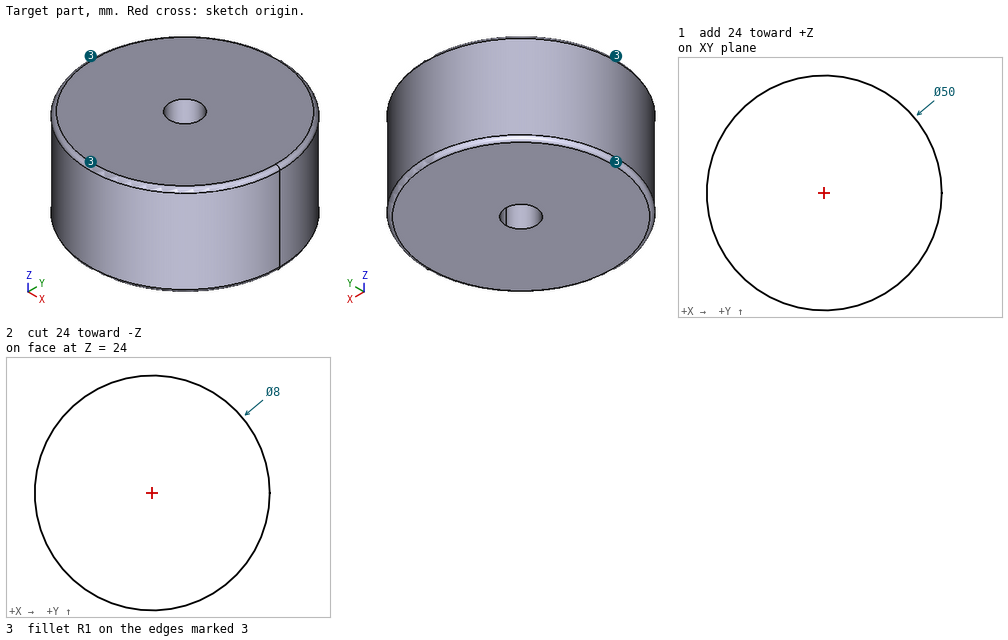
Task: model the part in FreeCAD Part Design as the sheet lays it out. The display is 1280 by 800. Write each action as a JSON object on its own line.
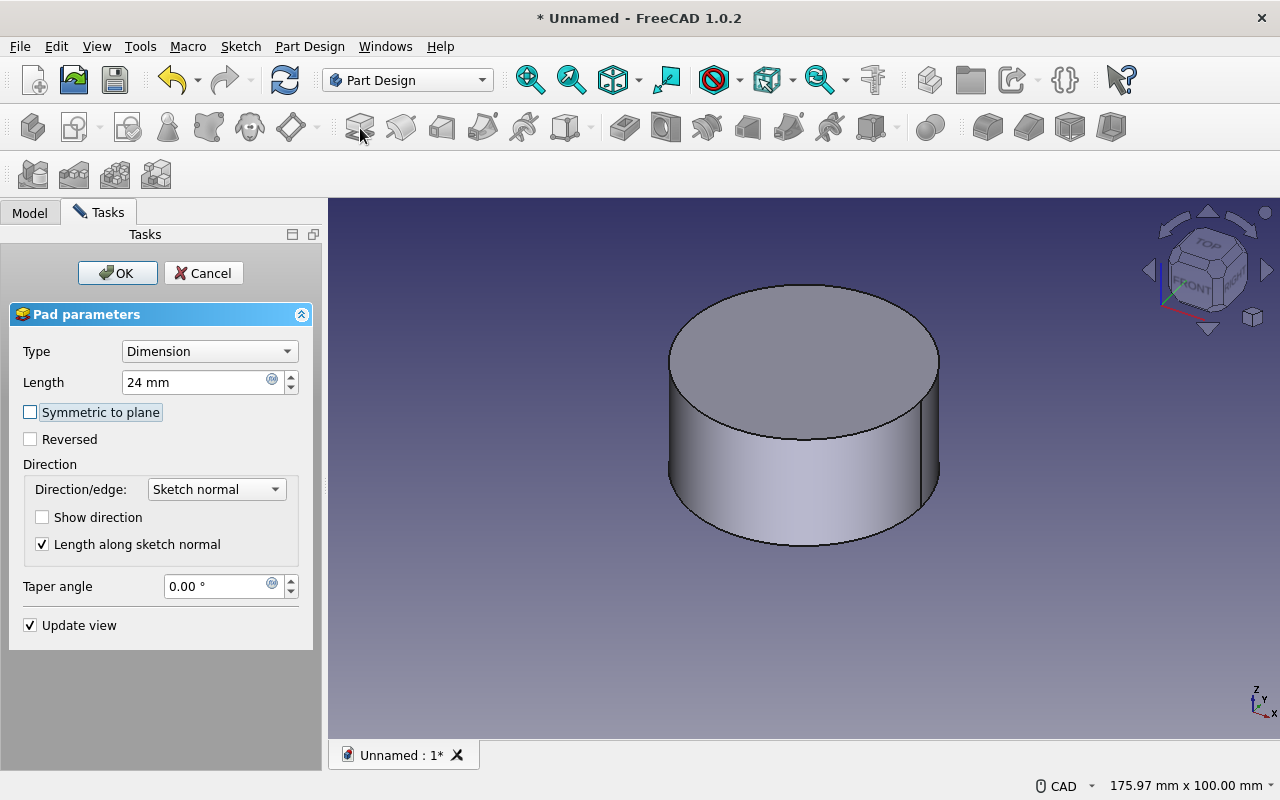
{"action": "left_click", "coordinate": [118, 273]}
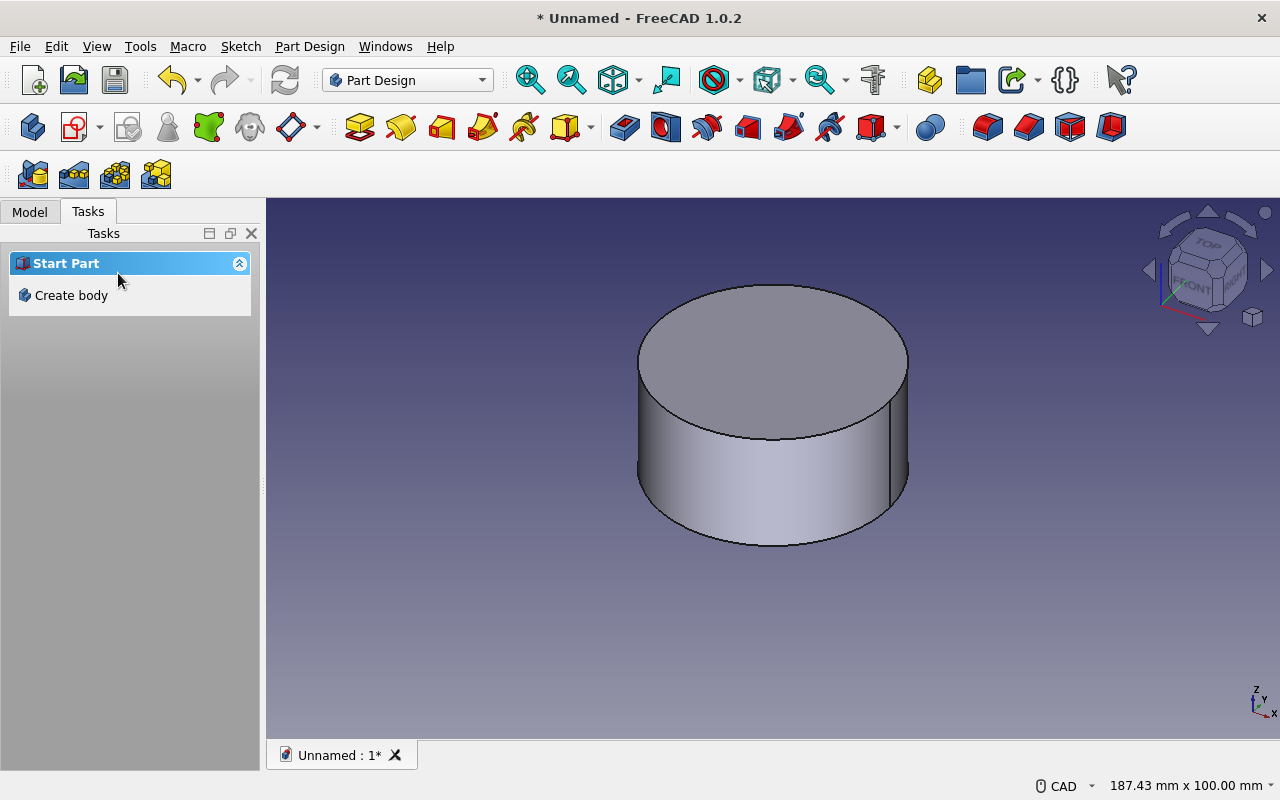
{"action": "left_click", "coordinate": [773, 361]}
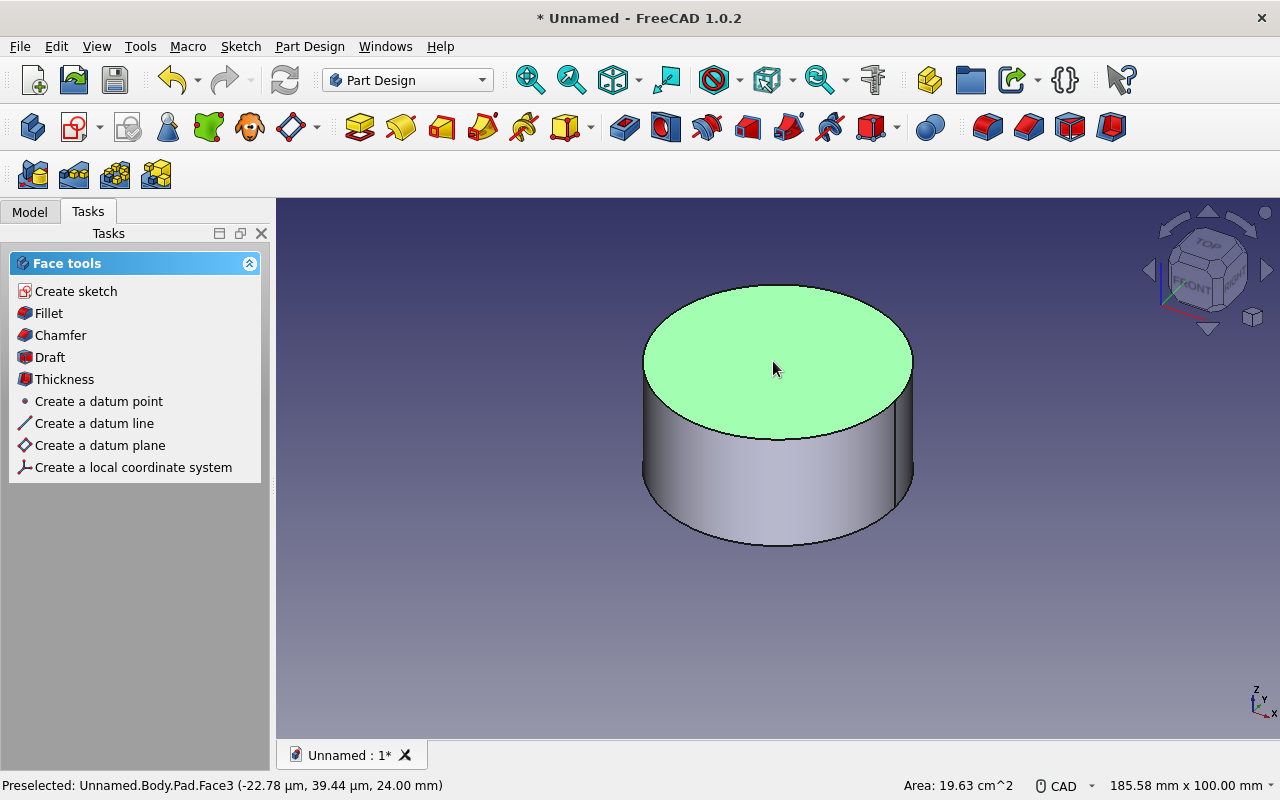
{"action": "left_click", "coordinate": [74, 128]}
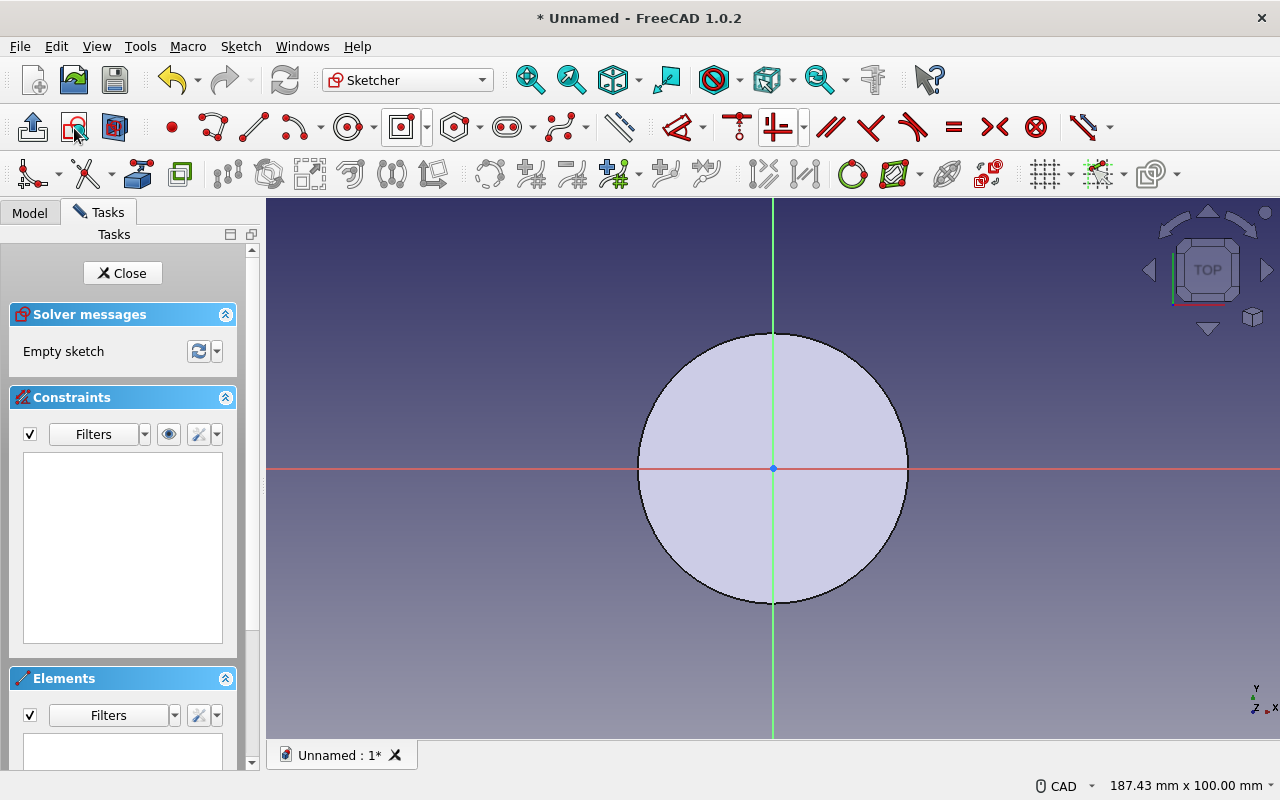
{"action": "scroll", "coordinate": [784, 468], "scroll_direction": "up", "scroll_amount": 10}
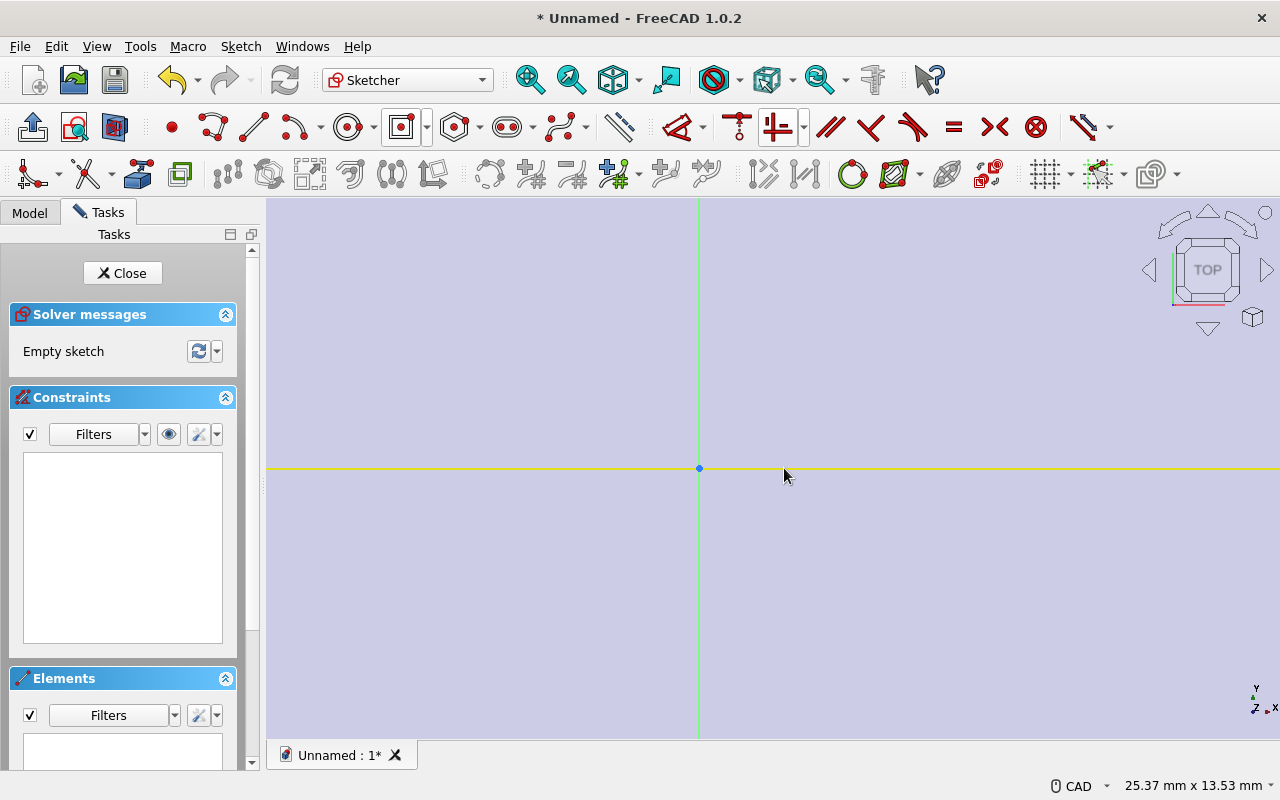
{"action": "key", "text": "g c"}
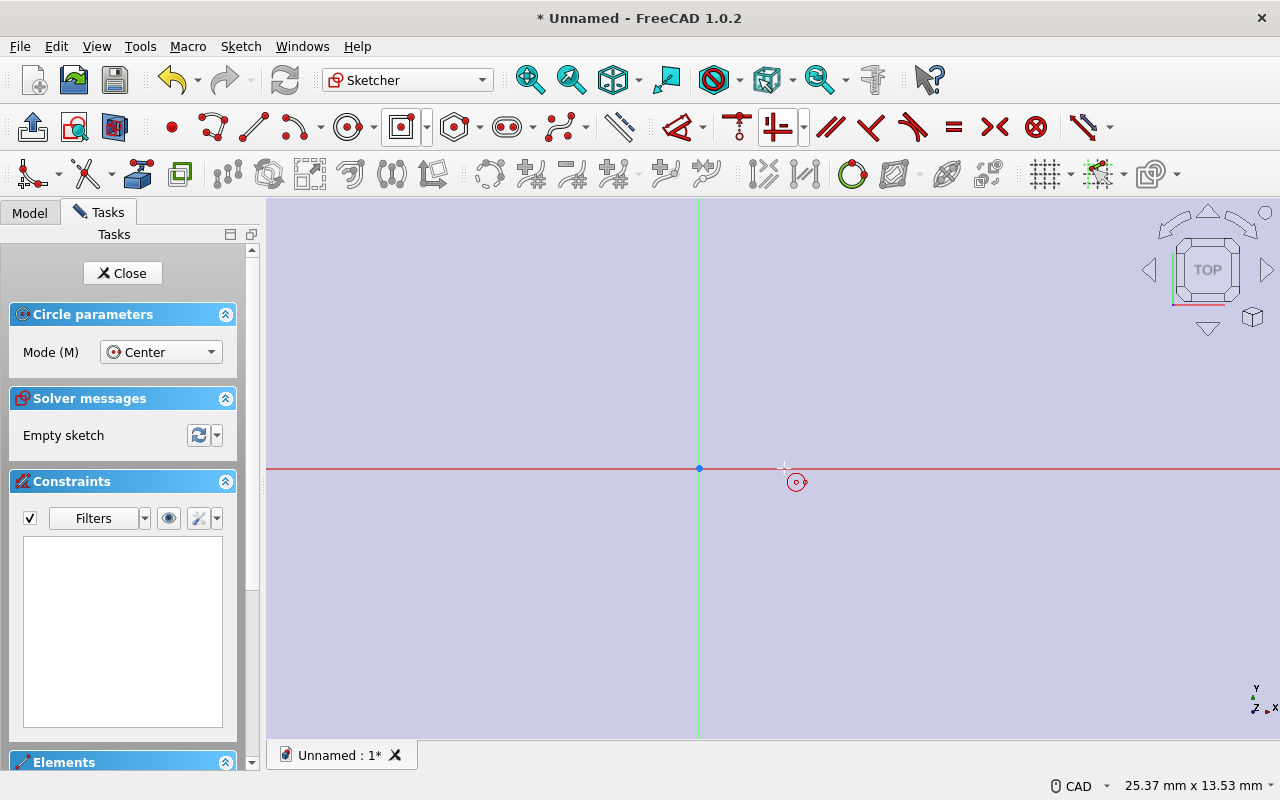
{"action": "left_click", "coordinate": [699, 468]}
{"action": "mouse_move", "coordinate": [813, 355]}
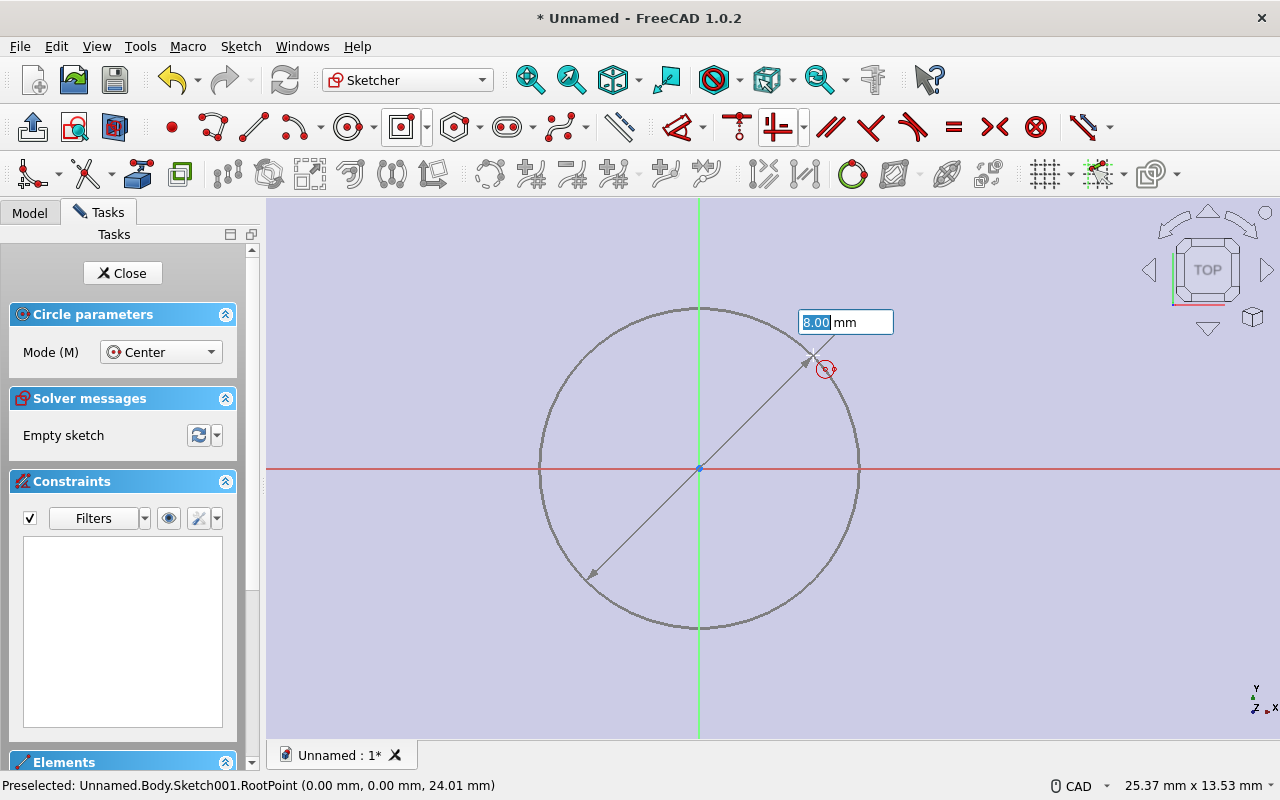
{"action": "type", "text": "8"}
{"action": "key", "text": "Return"}
{"action": "key", "text": "Escape"}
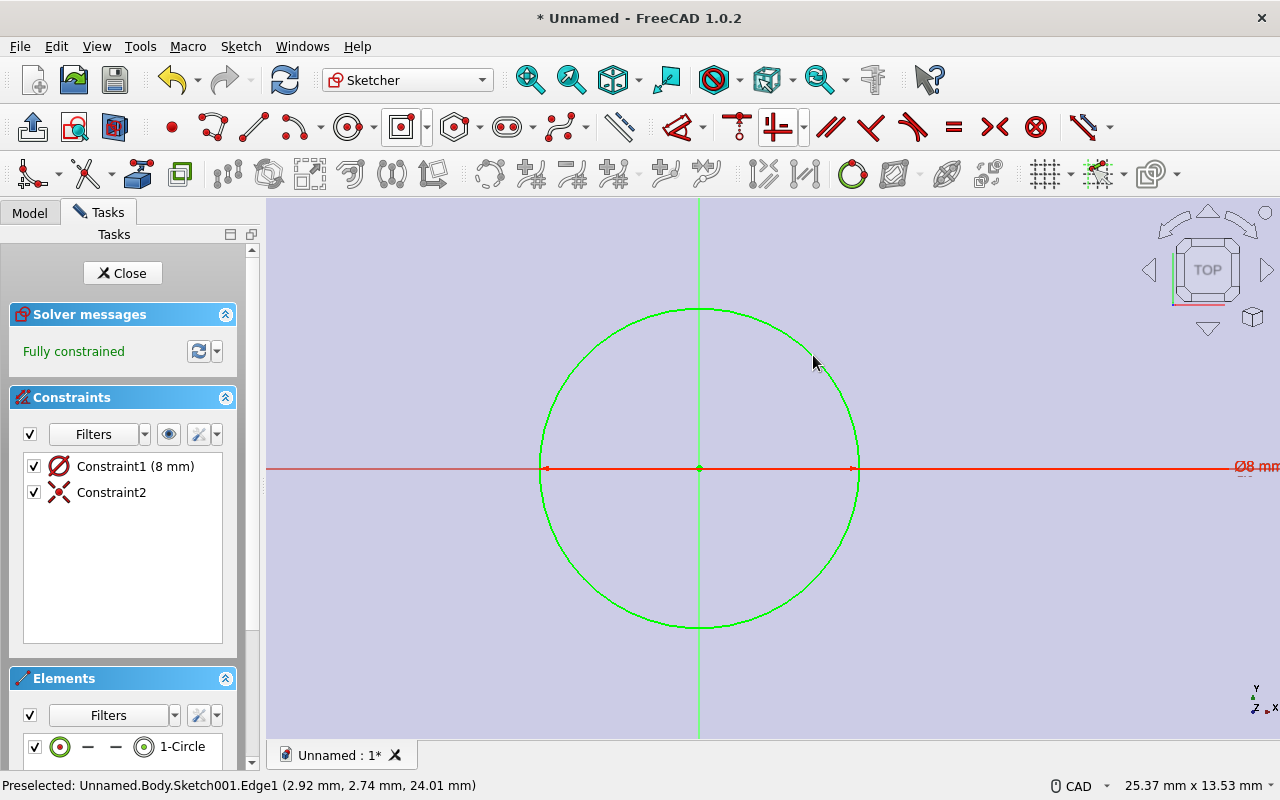
{"action": "left_click", "coordinate": [123, 273]}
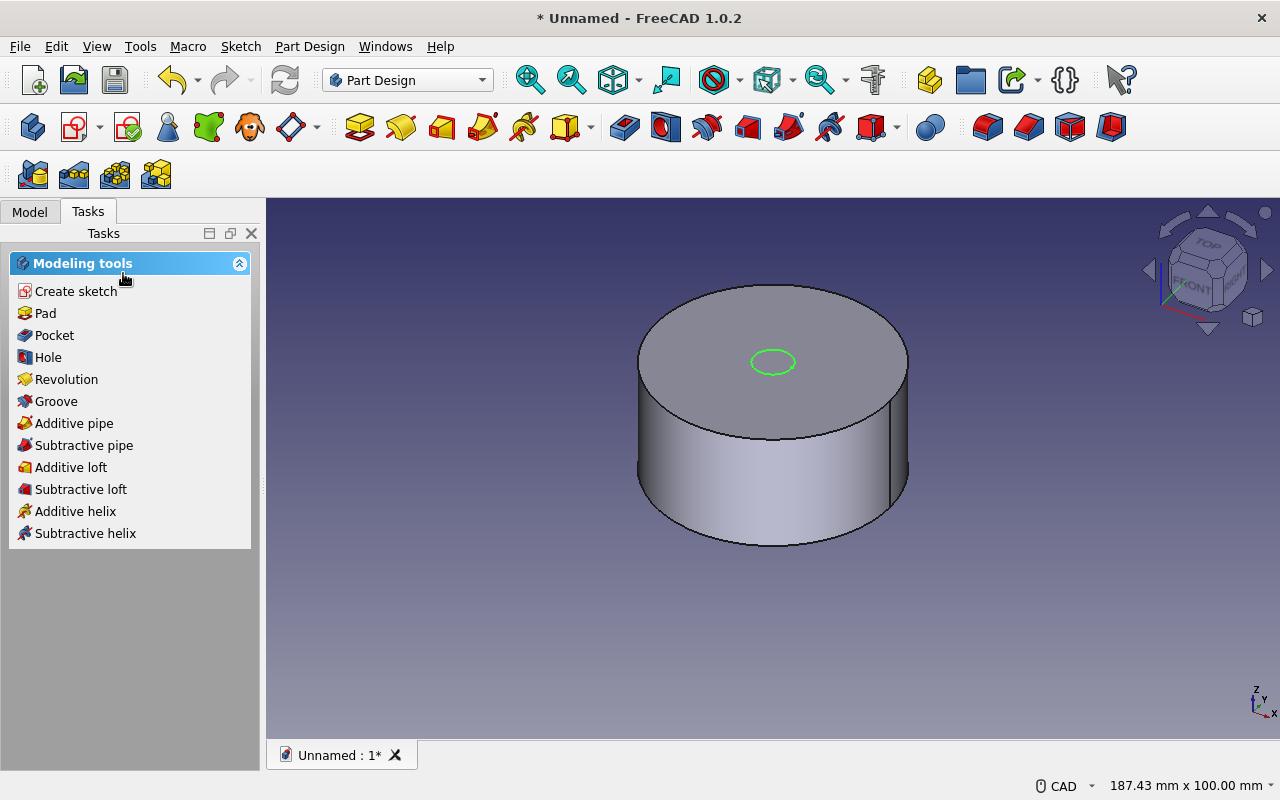
{"action": "left_click", "coordinate": [625, 128]}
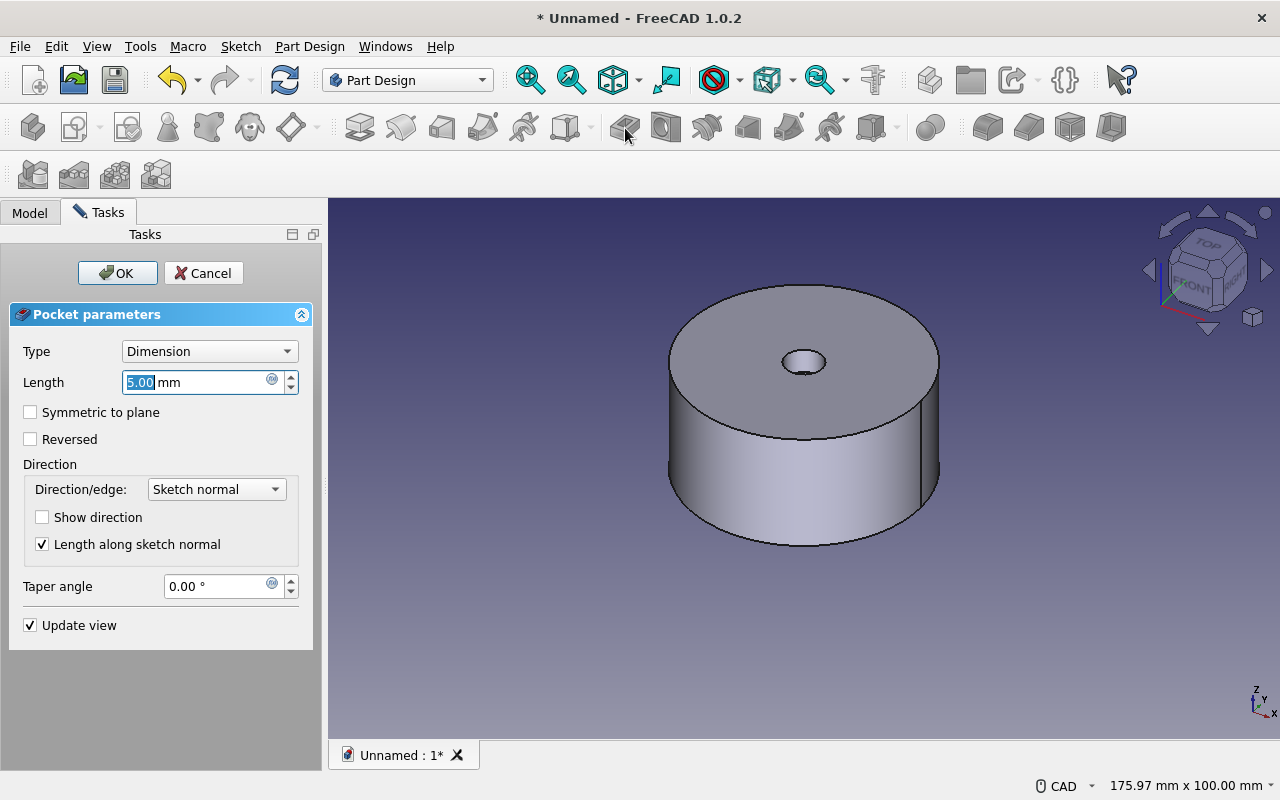
{"action": "type", "text": "24"}
{"action": "key", "text": "Tab"}